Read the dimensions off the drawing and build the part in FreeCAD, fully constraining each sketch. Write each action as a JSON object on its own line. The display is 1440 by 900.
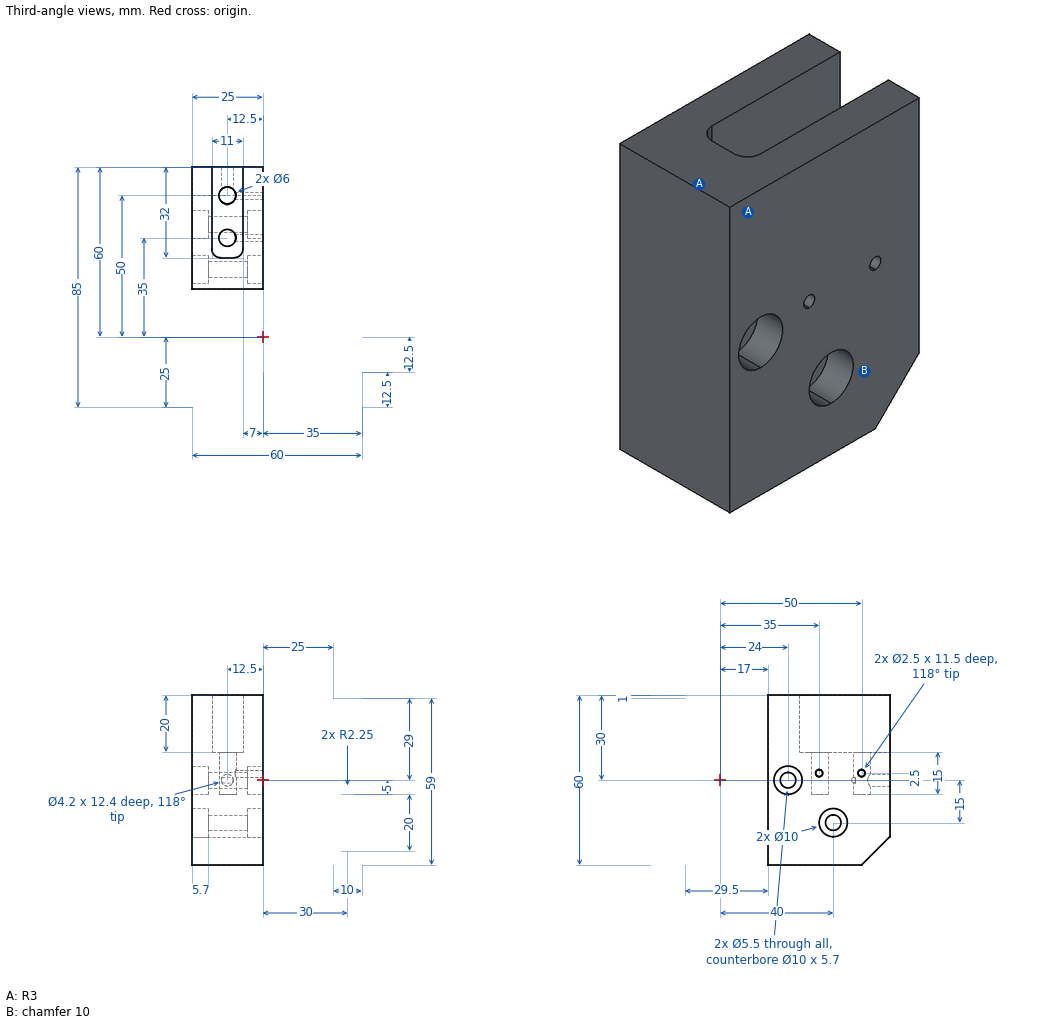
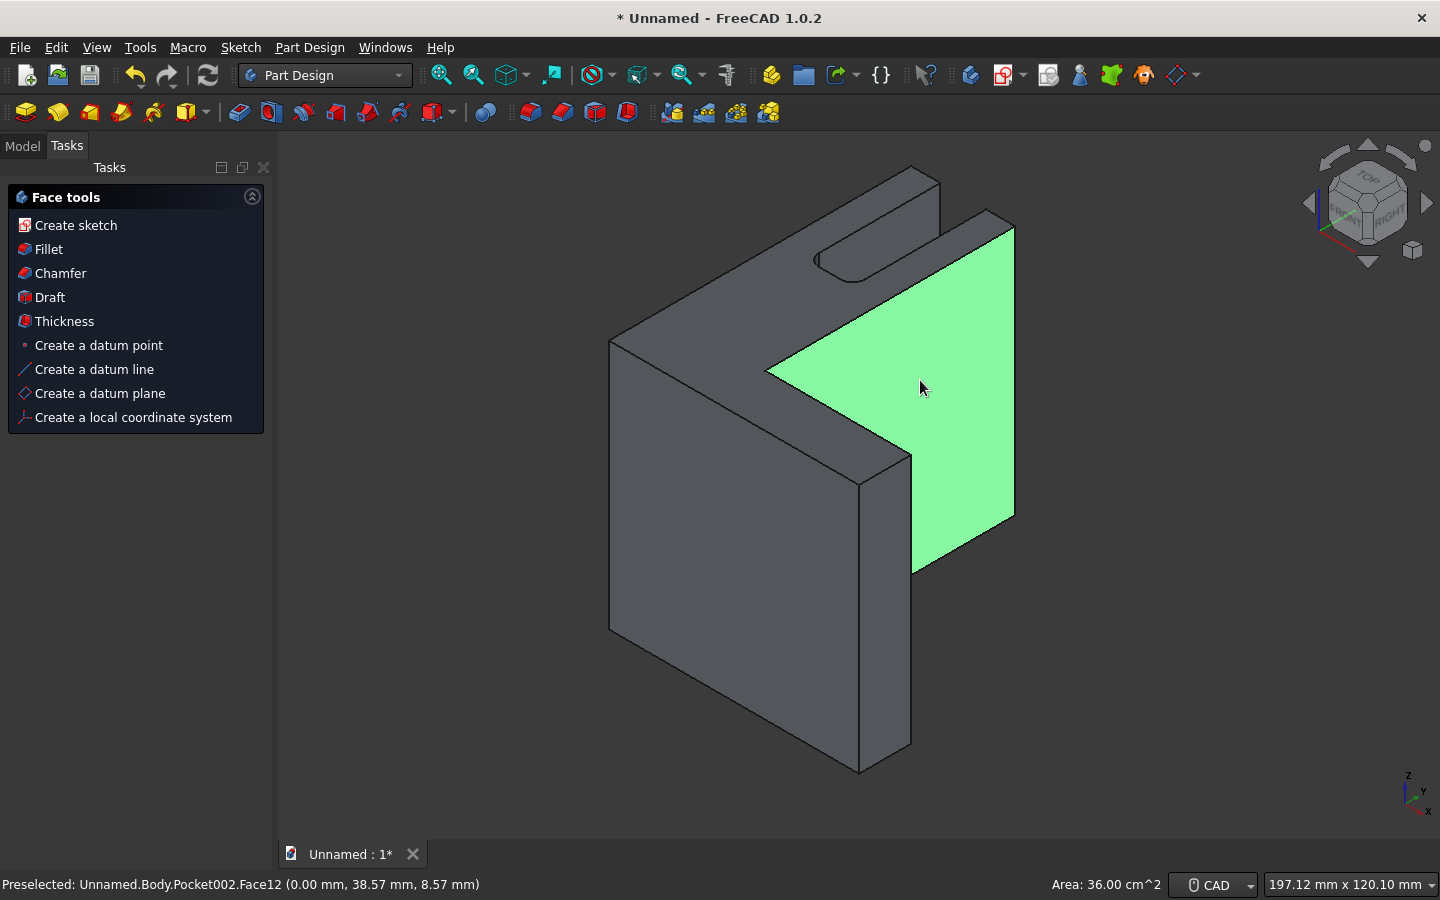
{"action": "left_click", "coordinate": [1004, 76]}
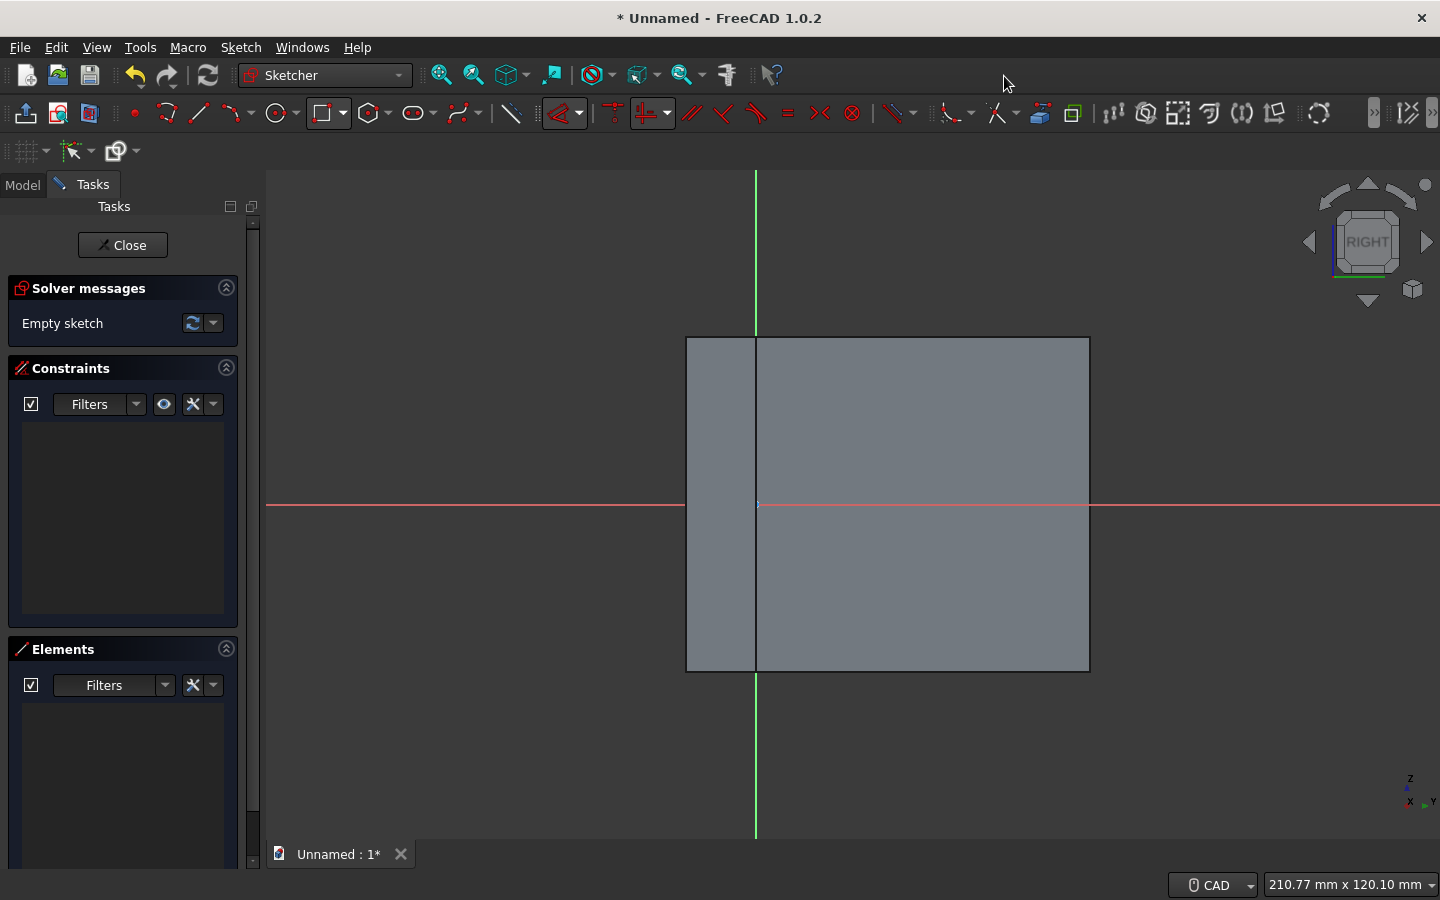
{"action": "scroll", "coordinate": [1025, 488], "scroll_direction": "up", "scroll_amount": 10}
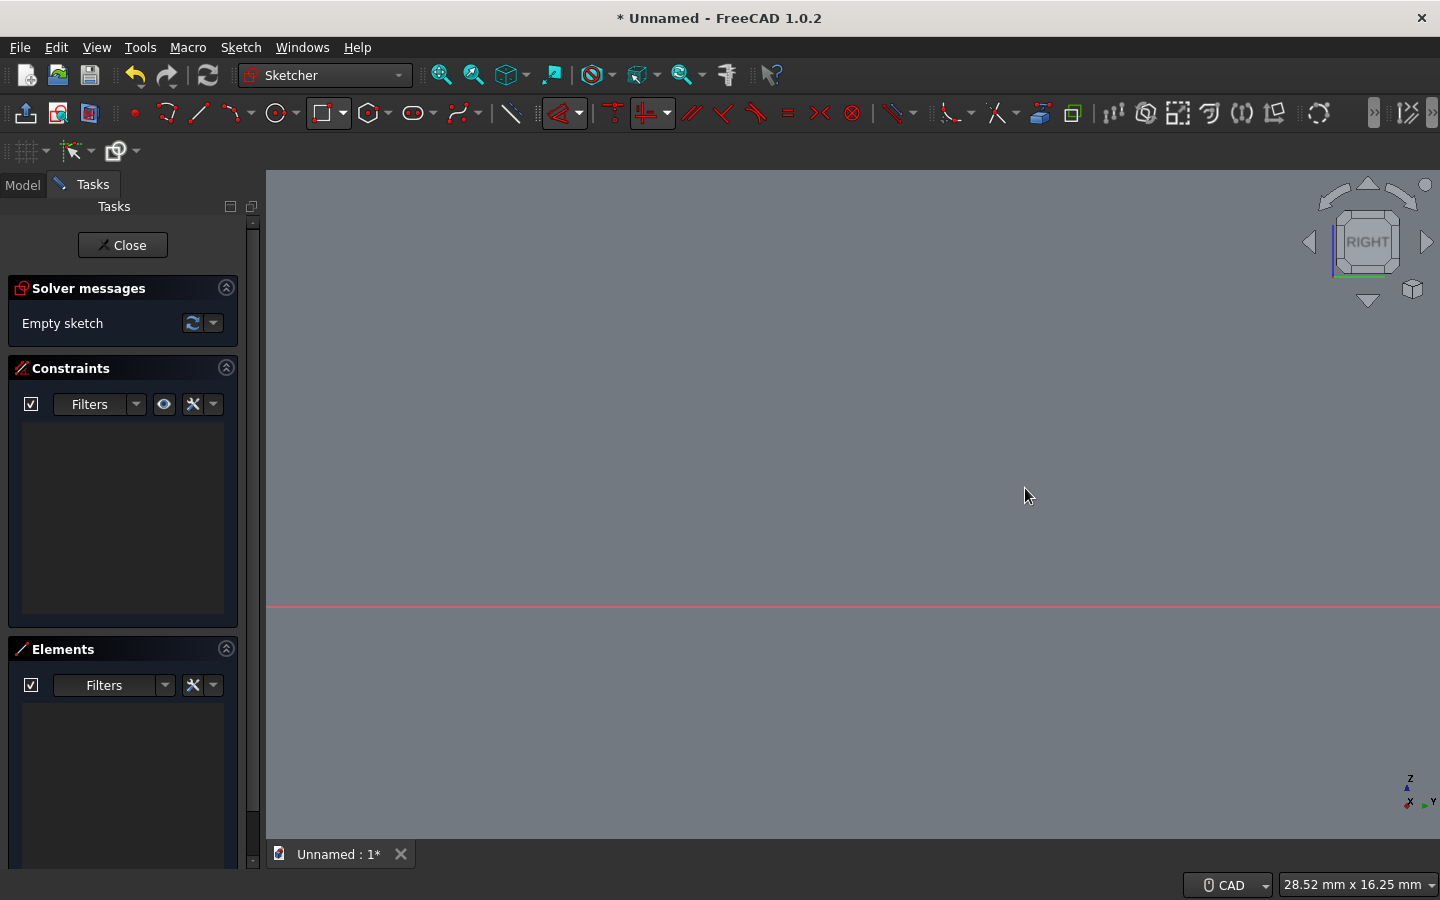
{"action": "left_click", "coordinate": [276, 114]}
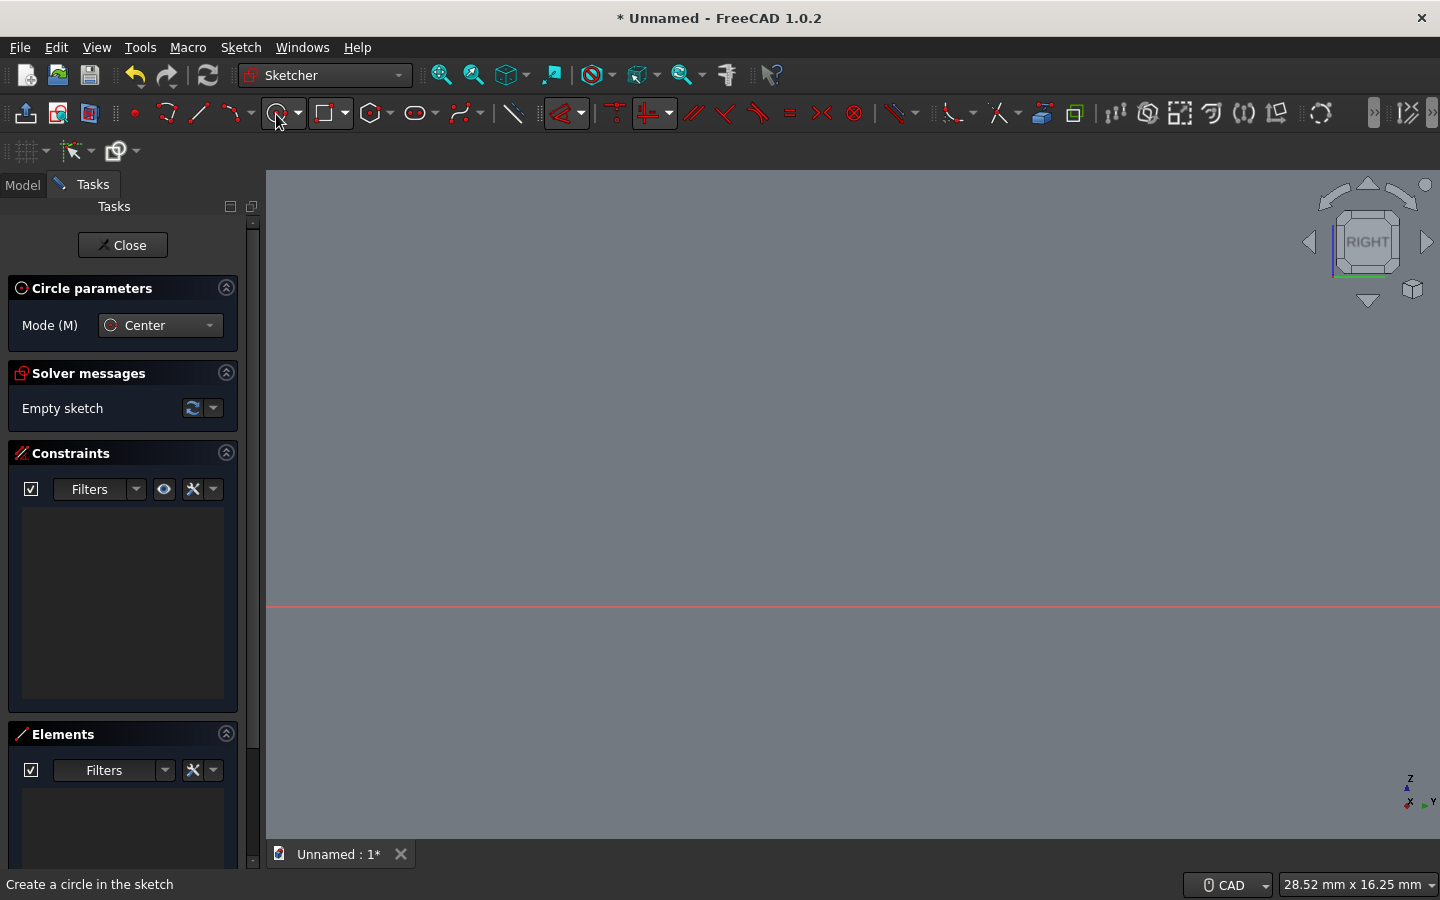
{"action": "left_click", "coordinate": [1088, 504]}
{"action": "mouse_move", "coordinate": [1124, 468]}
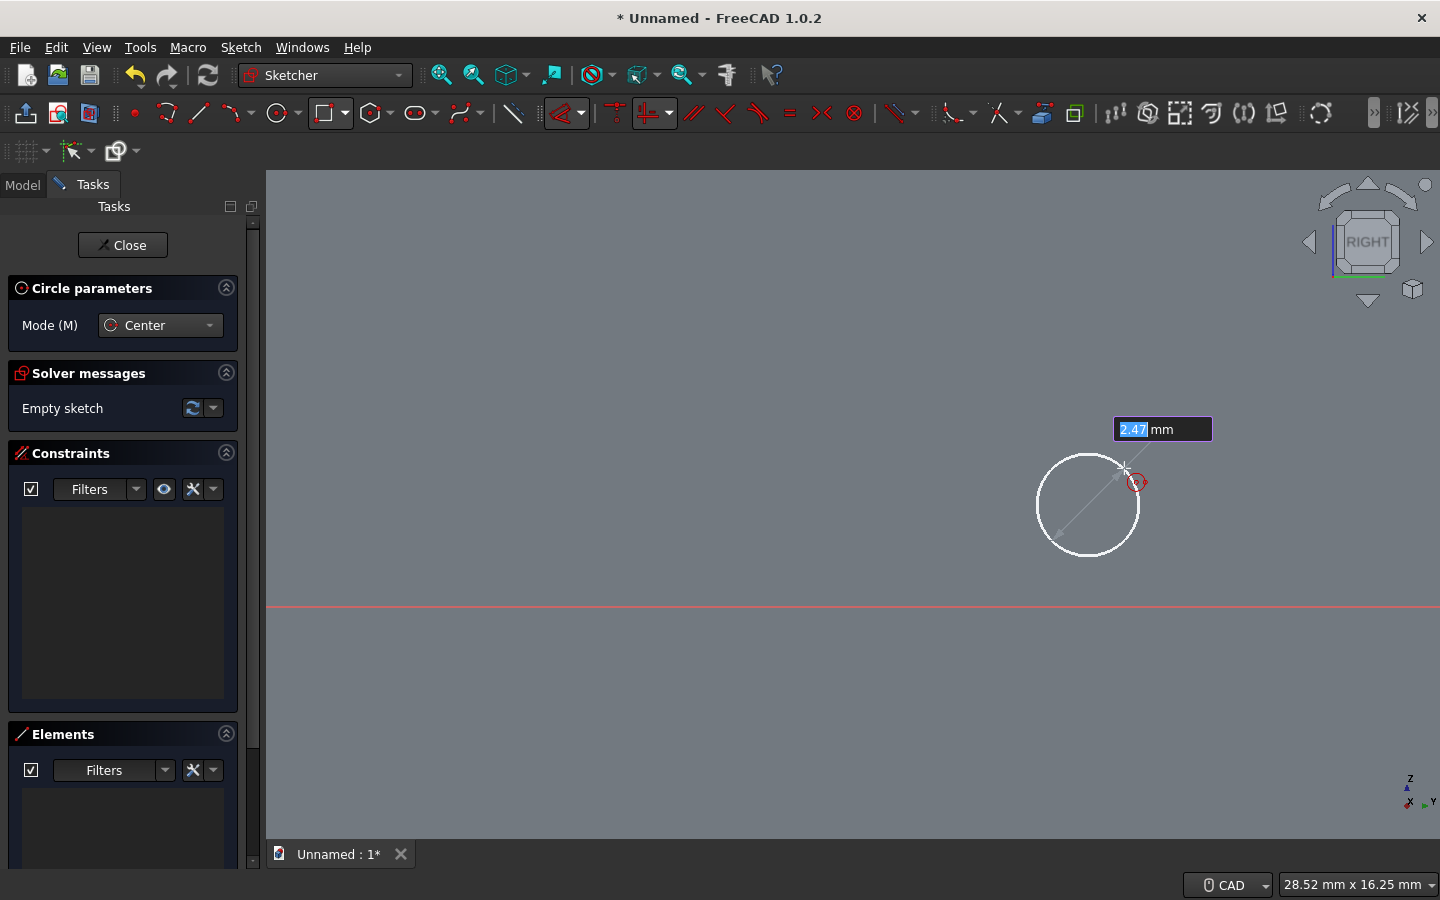
{"action": "type", "text": "2.5"}
{"action": "key", "text": "Return"}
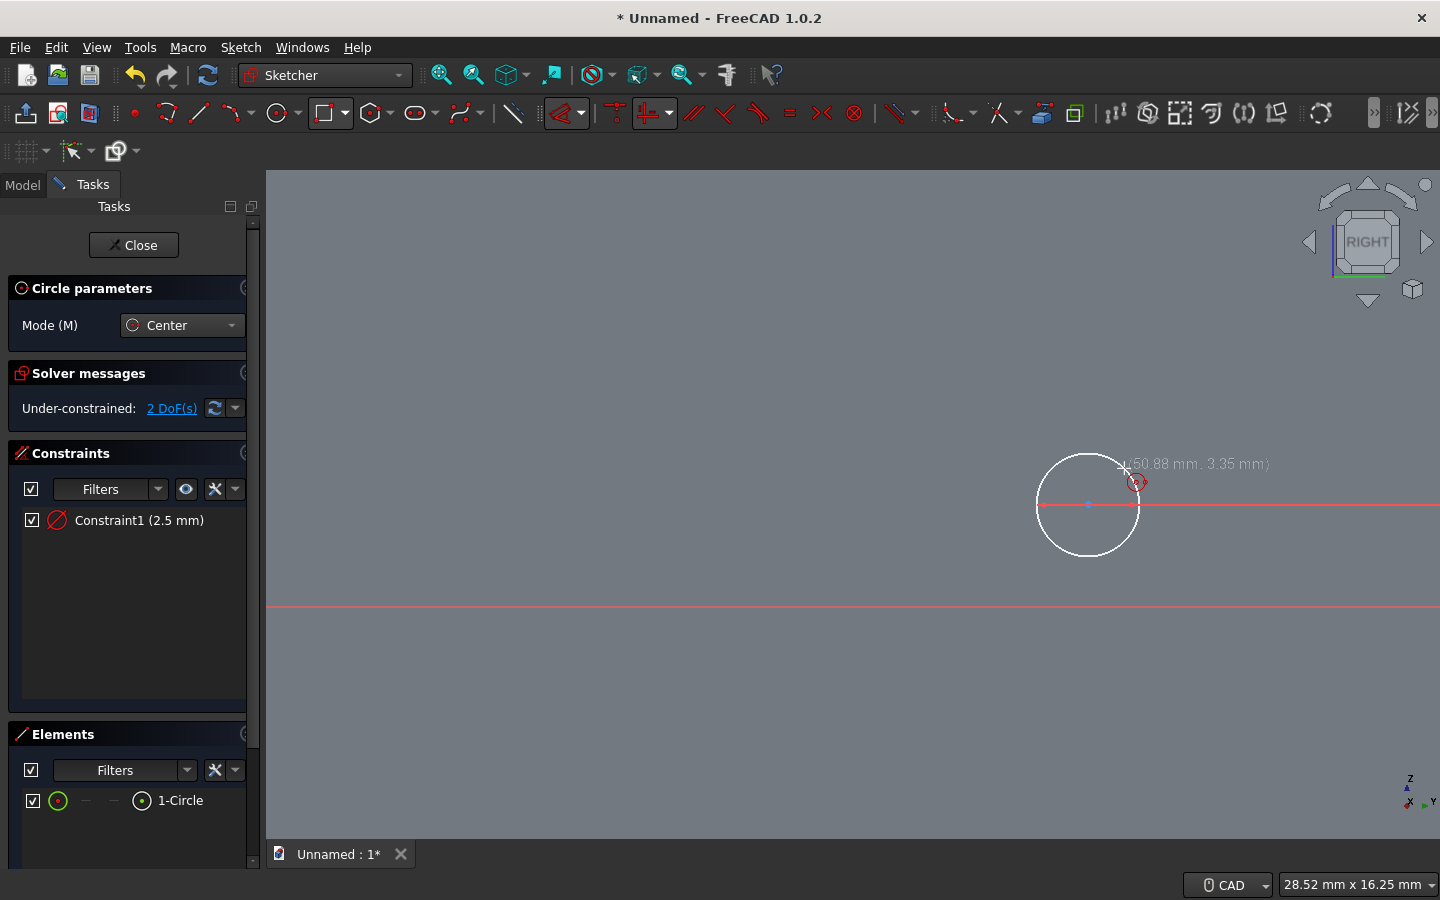
{"action": "left_click", "coordinate": [470, 504]}
{"action": "mouse_move", "coordinate": [507, 468]}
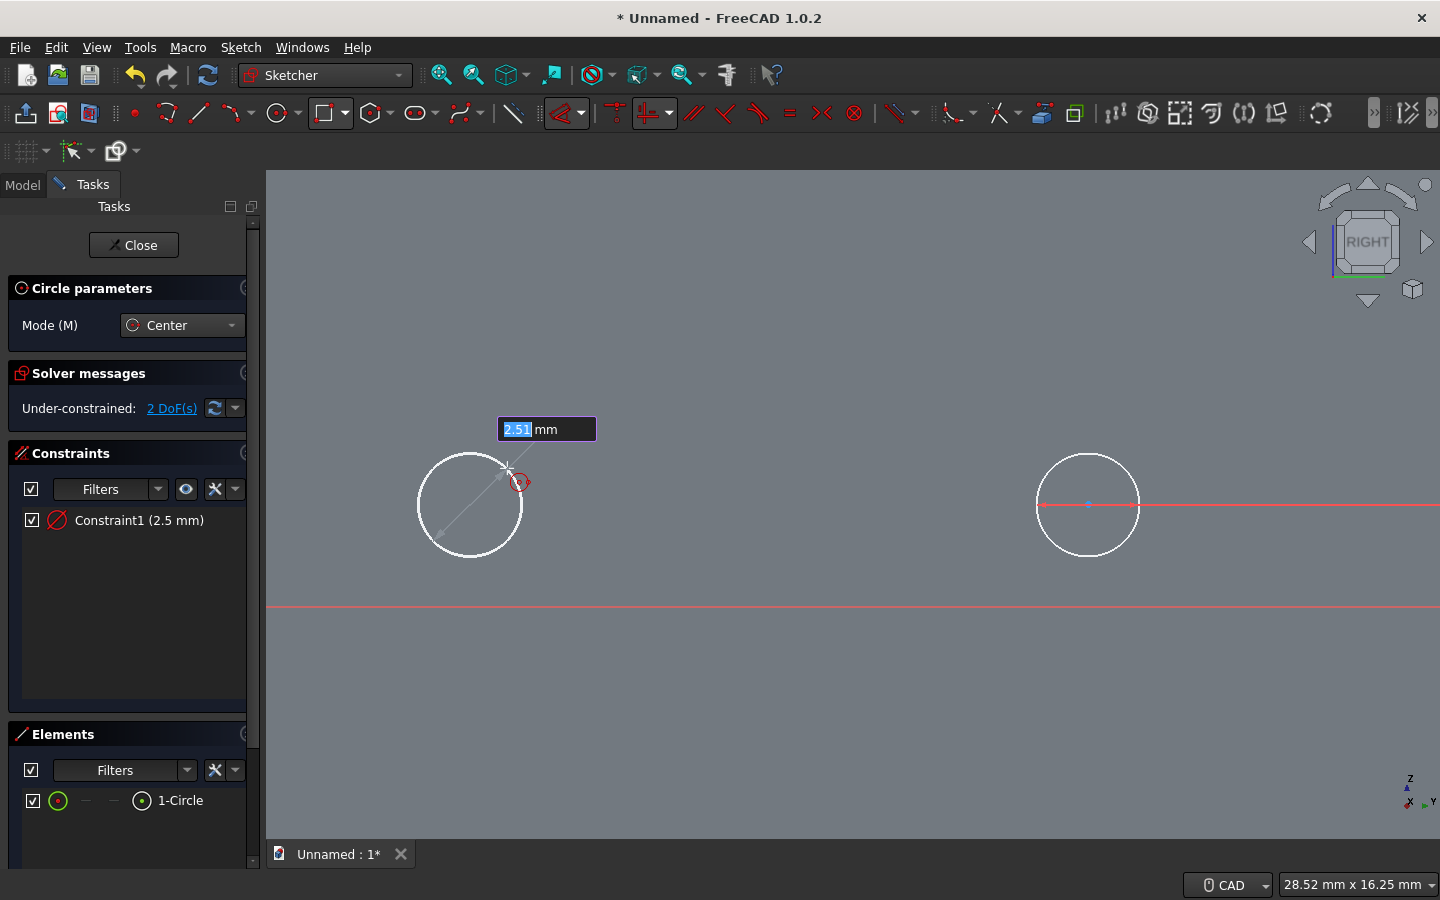
{"action": "type", "text": "2.5"}
{"action": "key", "text": "Return"}
{"action": "key", "text": "Escape"}